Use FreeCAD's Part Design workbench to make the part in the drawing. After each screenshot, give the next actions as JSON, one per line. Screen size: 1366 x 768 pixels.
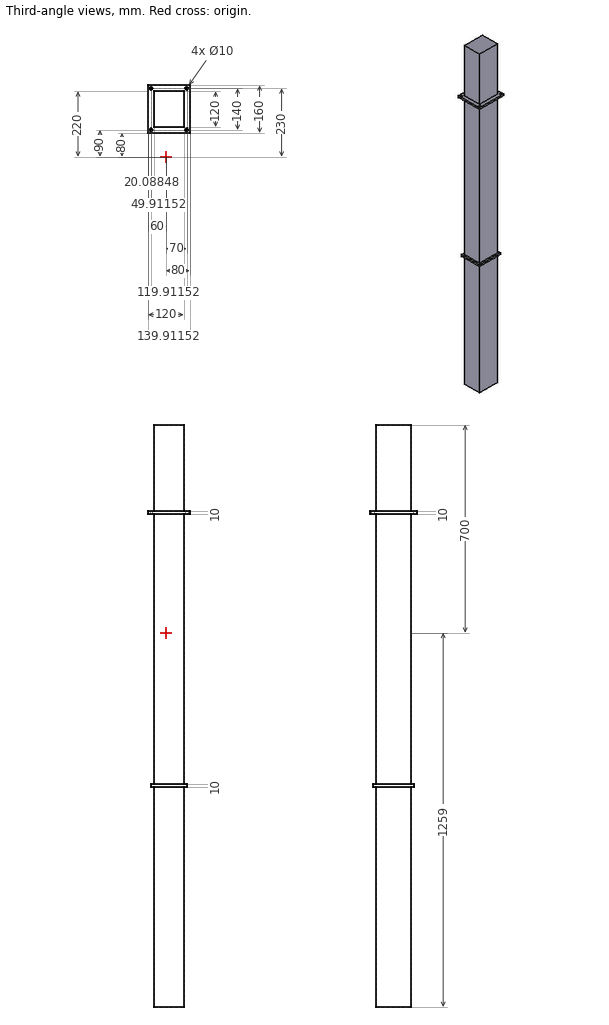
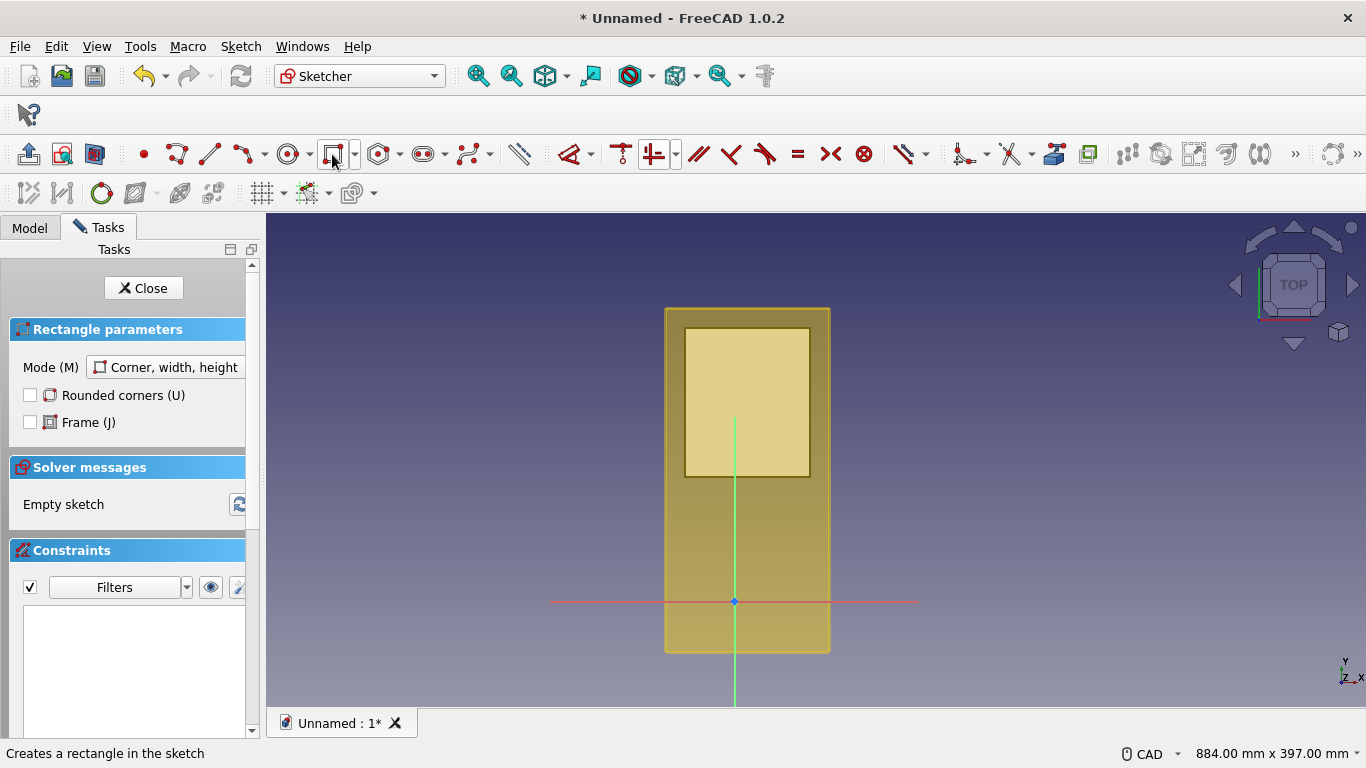
{"action": "left_click", "coordinate": [673, 315]}
{"action": "mouse_move", "coordinate": [822, 490]}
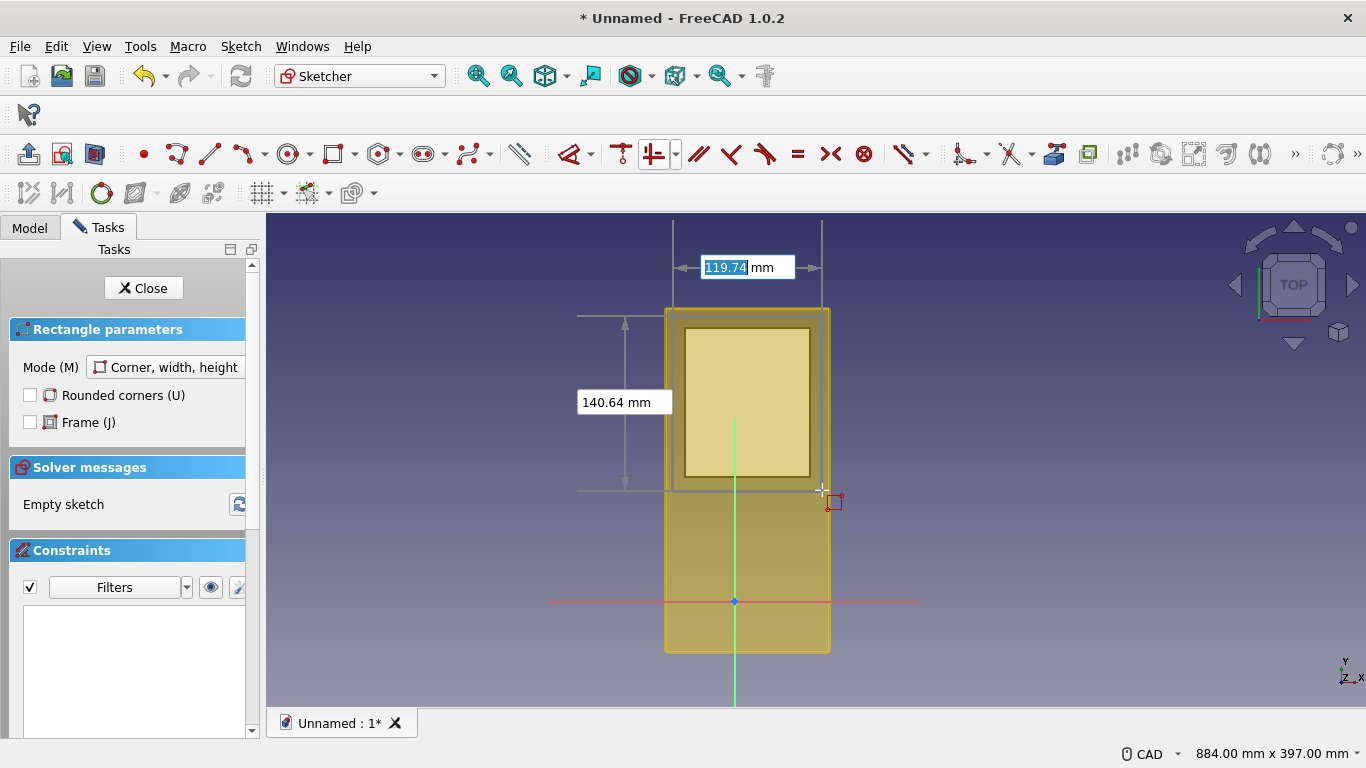
{"action": "type", "text": "119.91152"}
{"action": "key", "text": "Tab"}
{"action": "type", "text": "140"}
{"action": "key", "text": "Return"}
{"action": "key", "text": "Escape"}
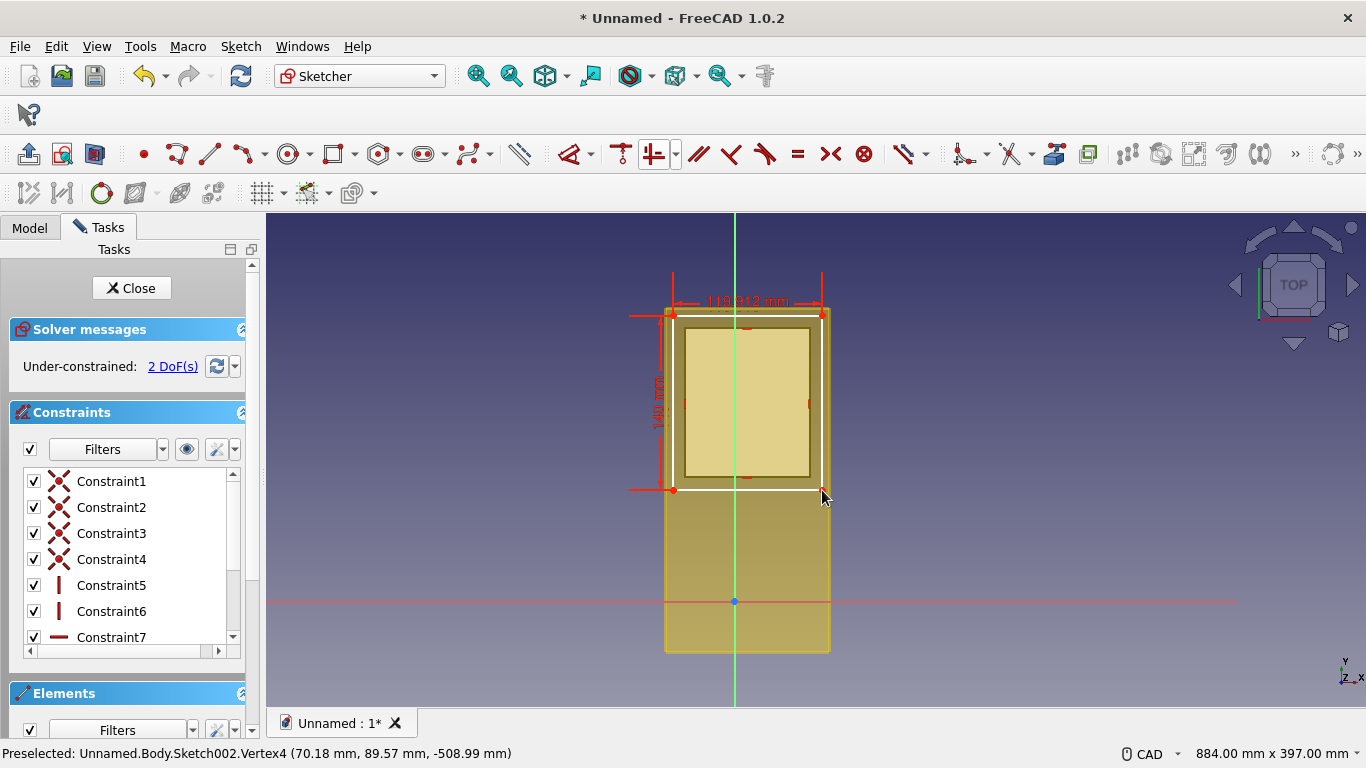
{"action": "key", "text": "d"}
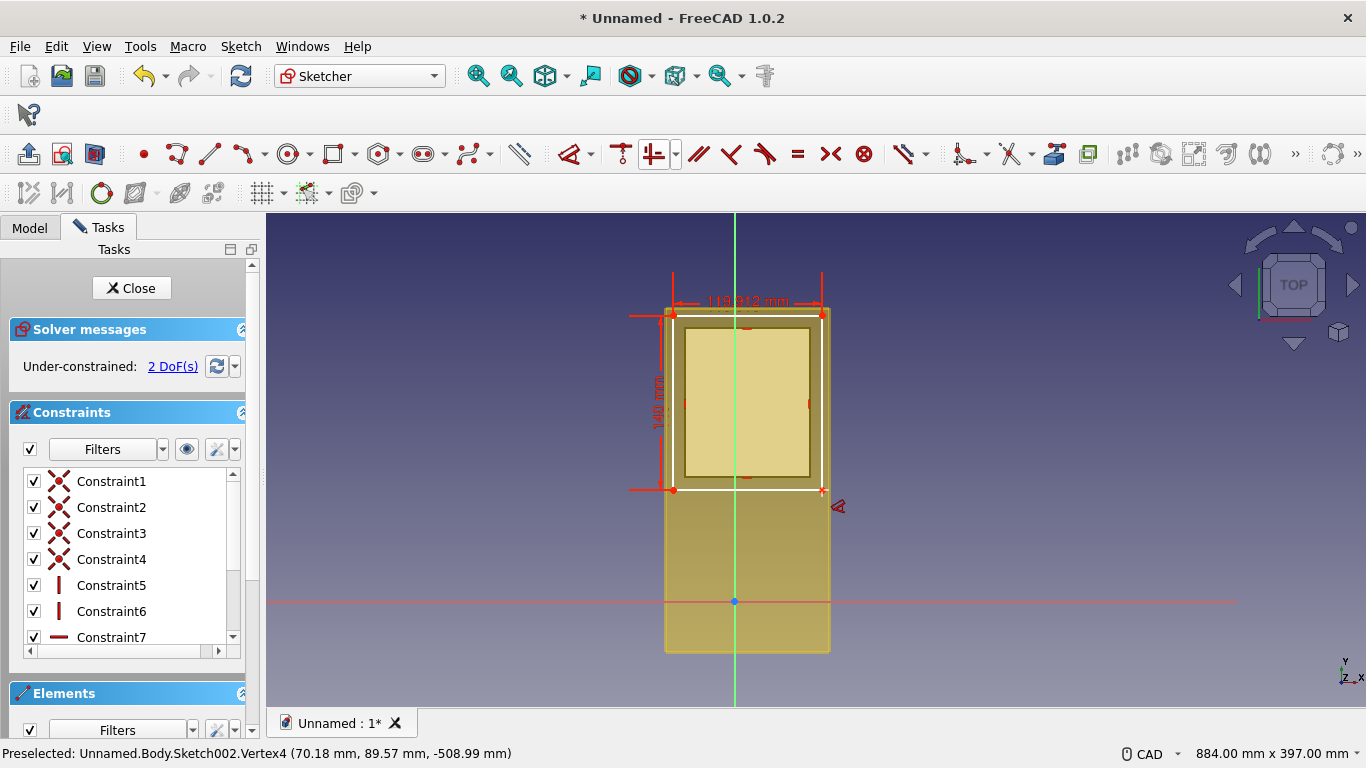
{"action": "left_click", "coordinate": [673, 490]}
{"action": "left_click", "coordinate": [639, 546]}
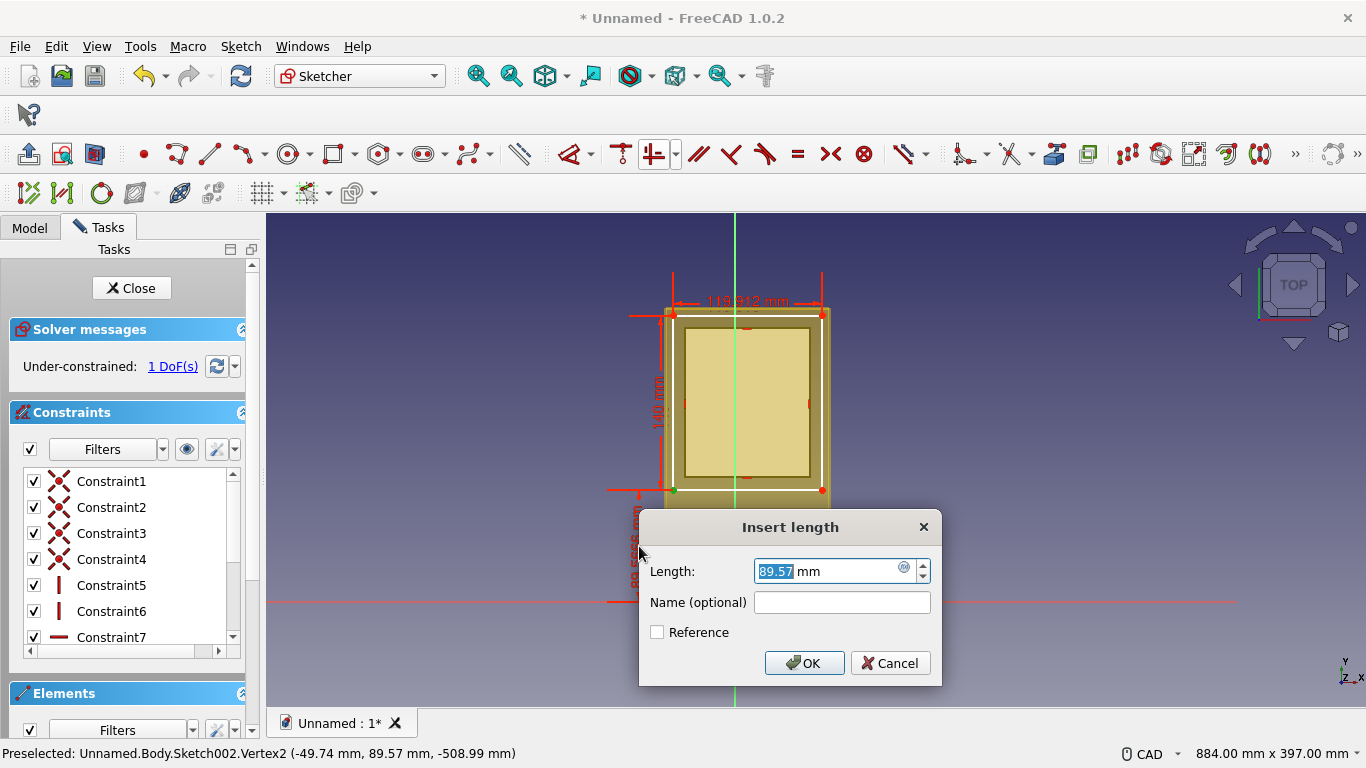
{"action": "type", "text": "90"}
{"action": "key", "text": "Return"}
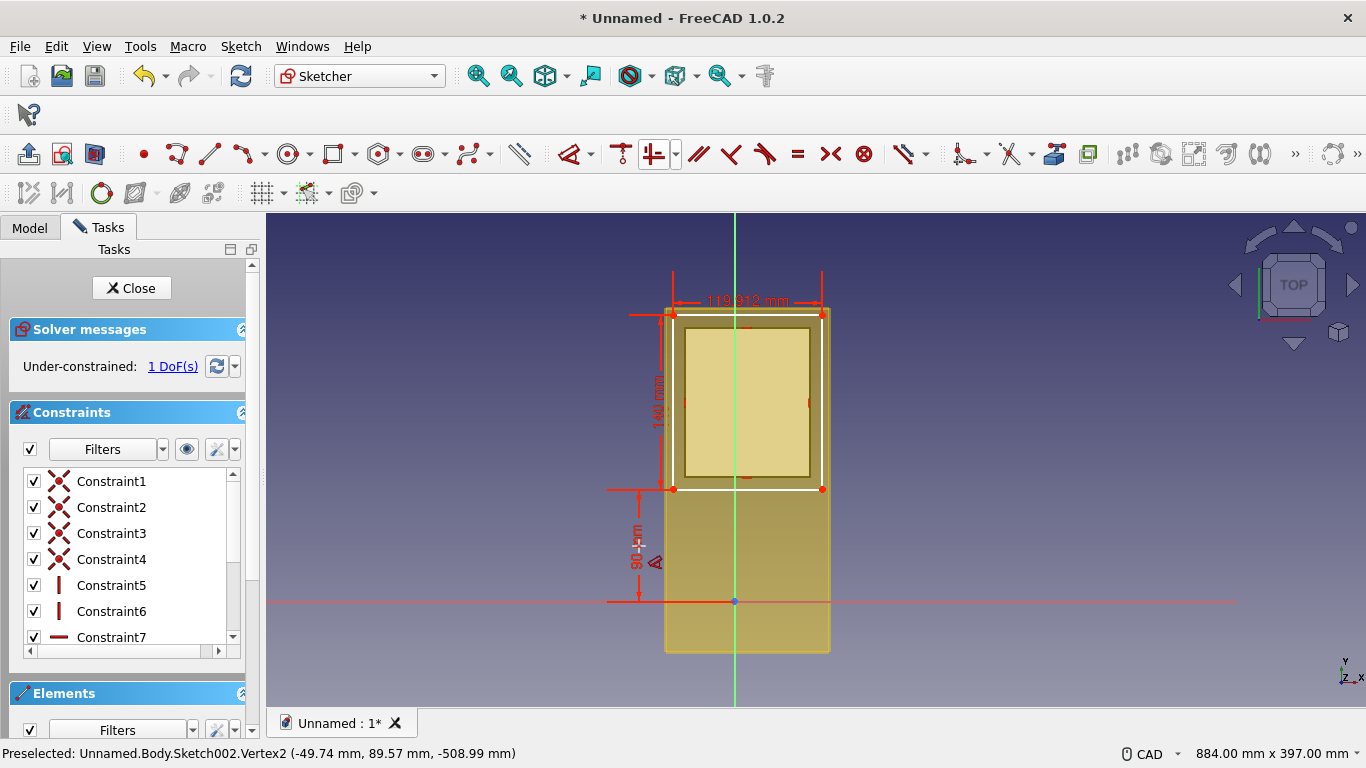
{"action": "left_click", "coordinate": [822, 490]}
{"action": "left_click", "coordinate": [779, 636]}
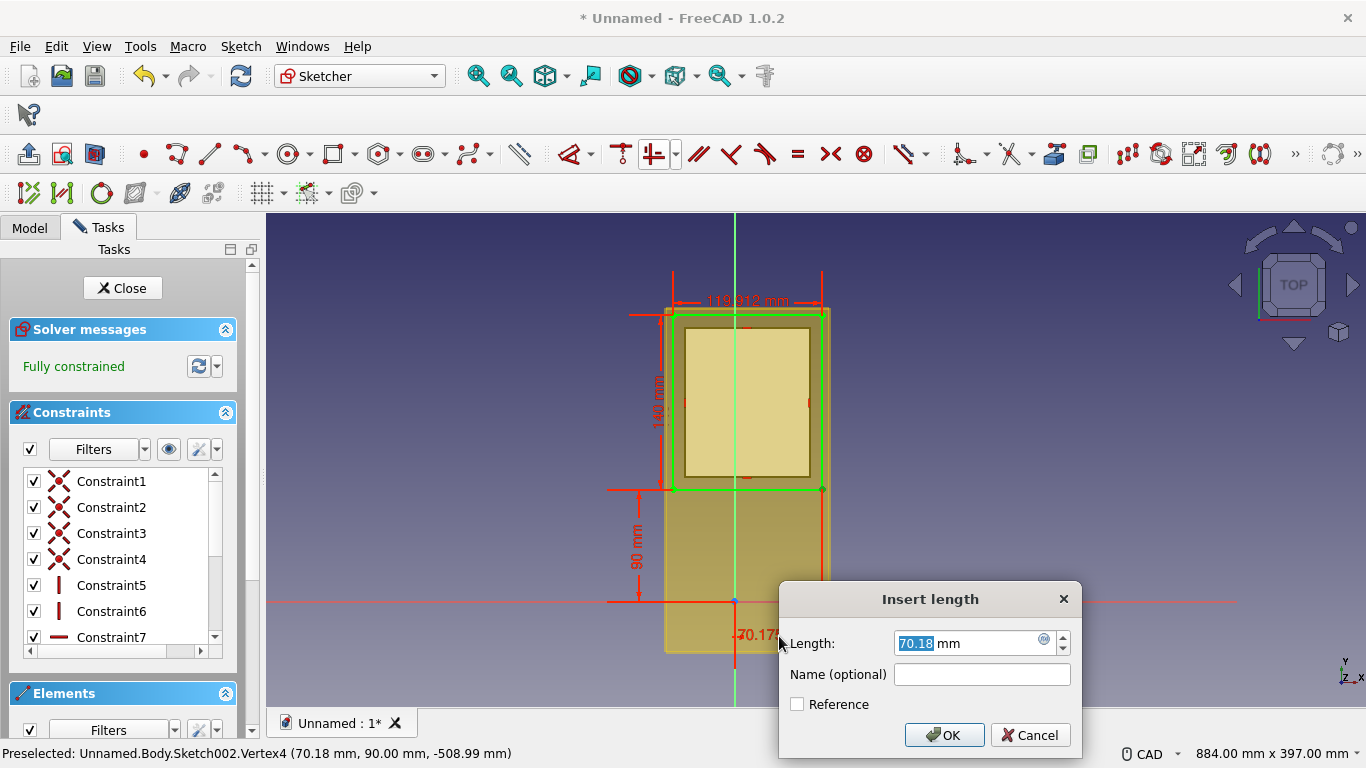
{"action": "type", "text": "70"}
{"action": "key", "text": "Return"}
{"action": "key", "text": "Escape"}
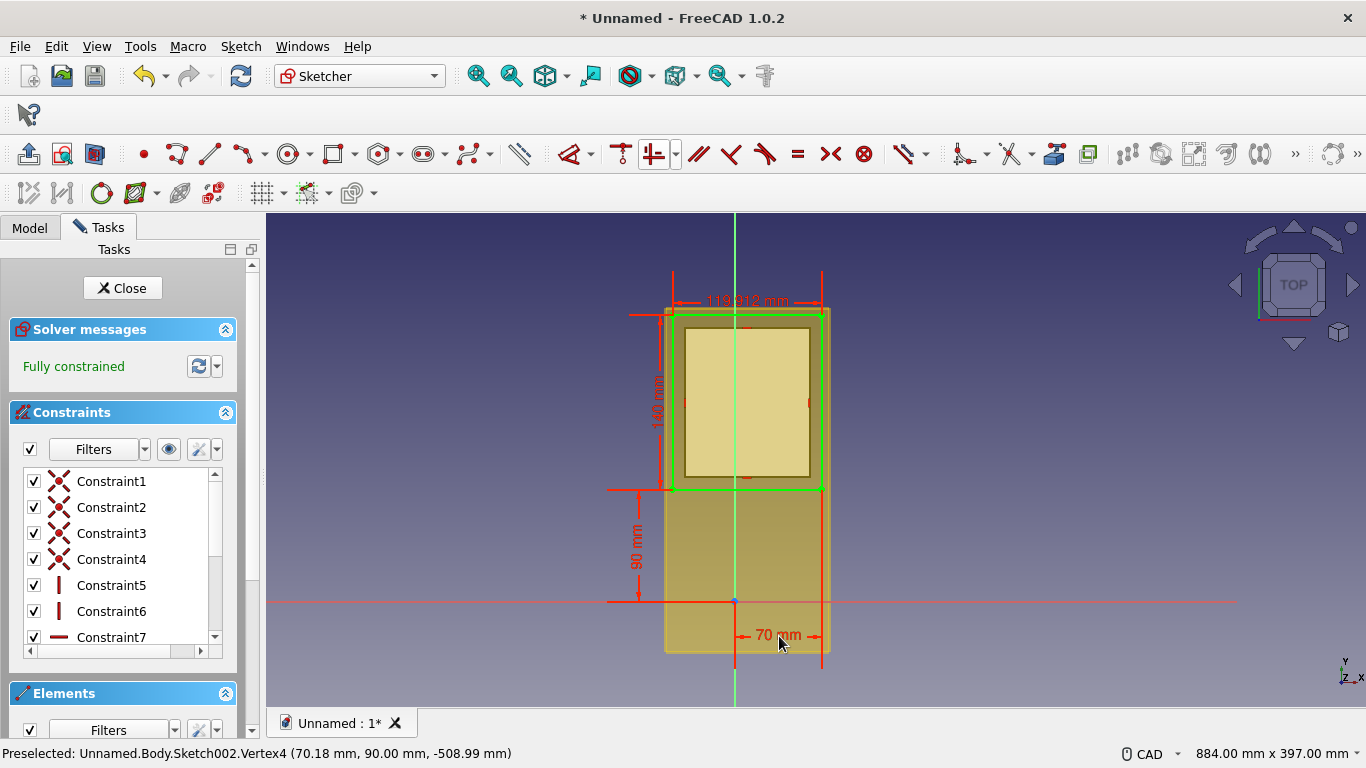
{"action": "left_click", "coordinate": [123, 288]}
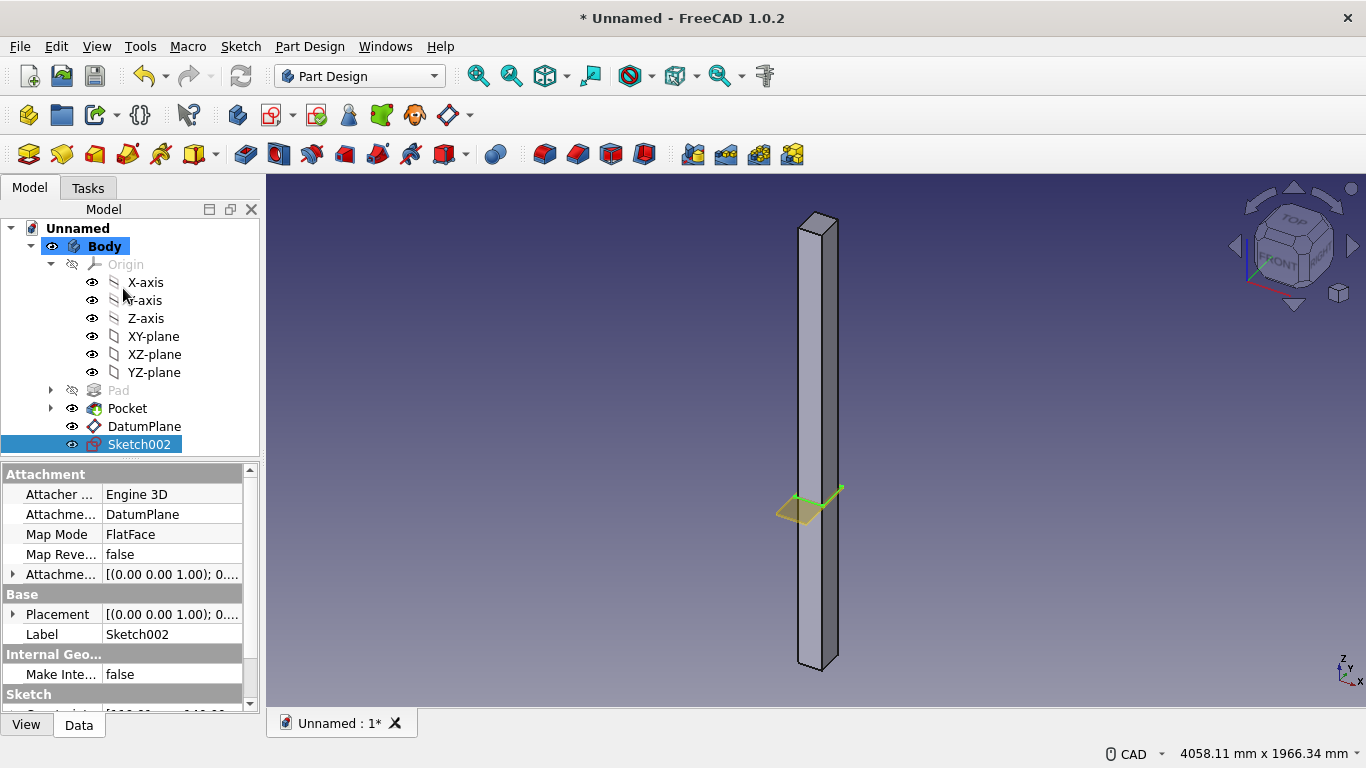
{"action": "left_click", "coordinate": [29, 154]}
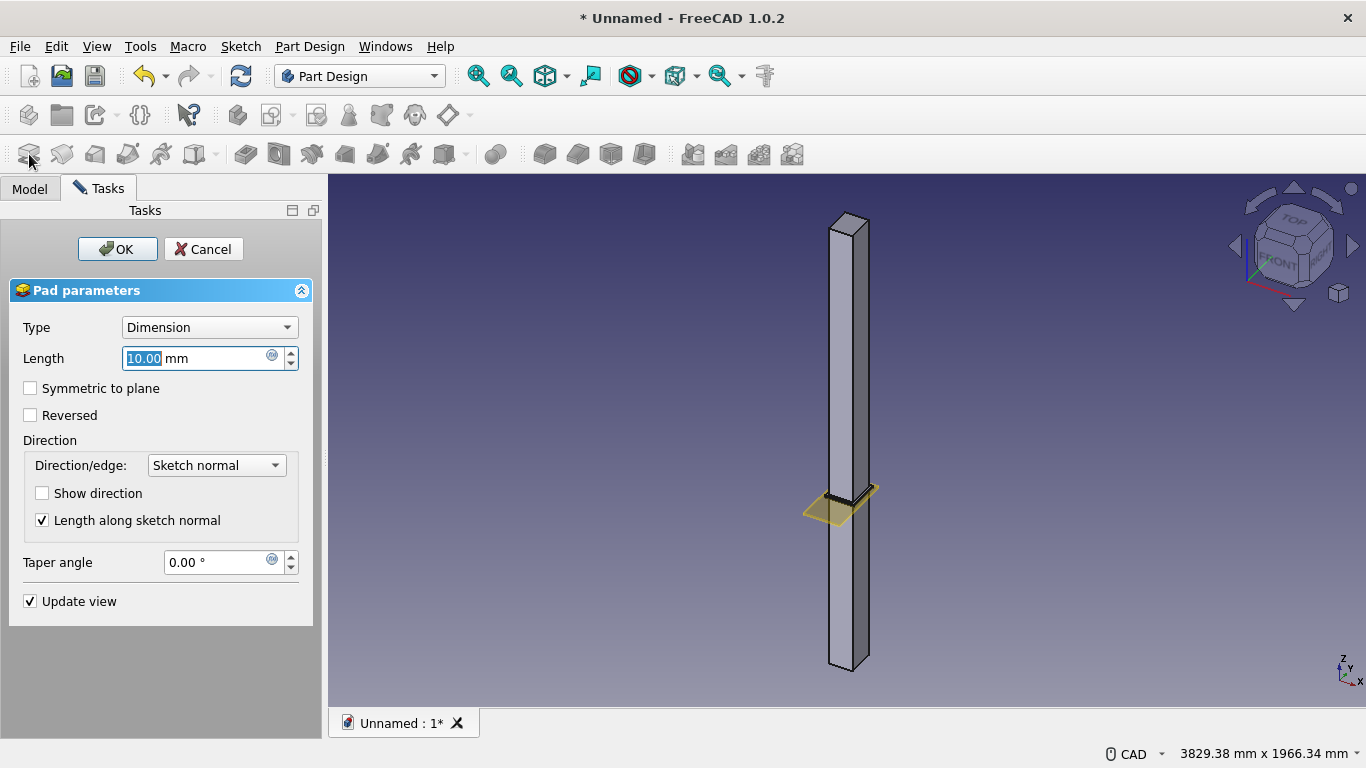
{"action": "type", "text": "10"}
{"action": "key", "text": "Tab"}